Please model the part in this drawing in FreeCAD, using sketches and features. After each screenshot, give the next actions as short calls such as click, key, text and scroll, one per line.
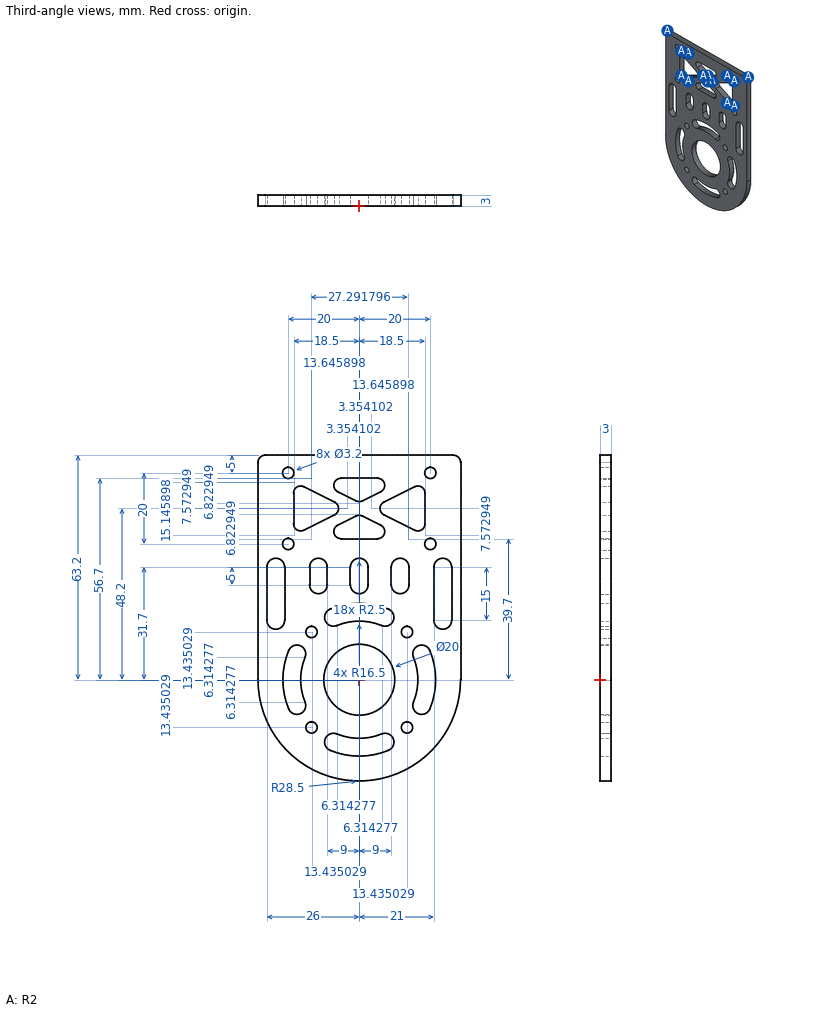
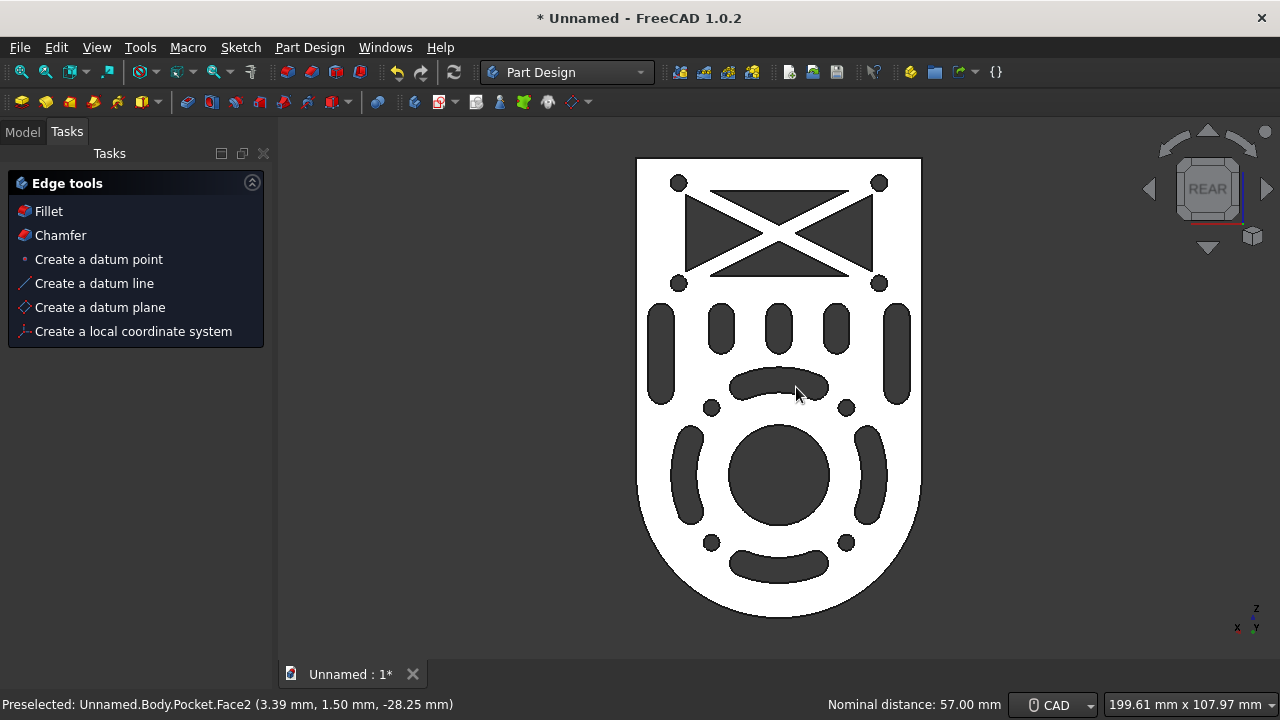
scroll(762, 232, up, 5)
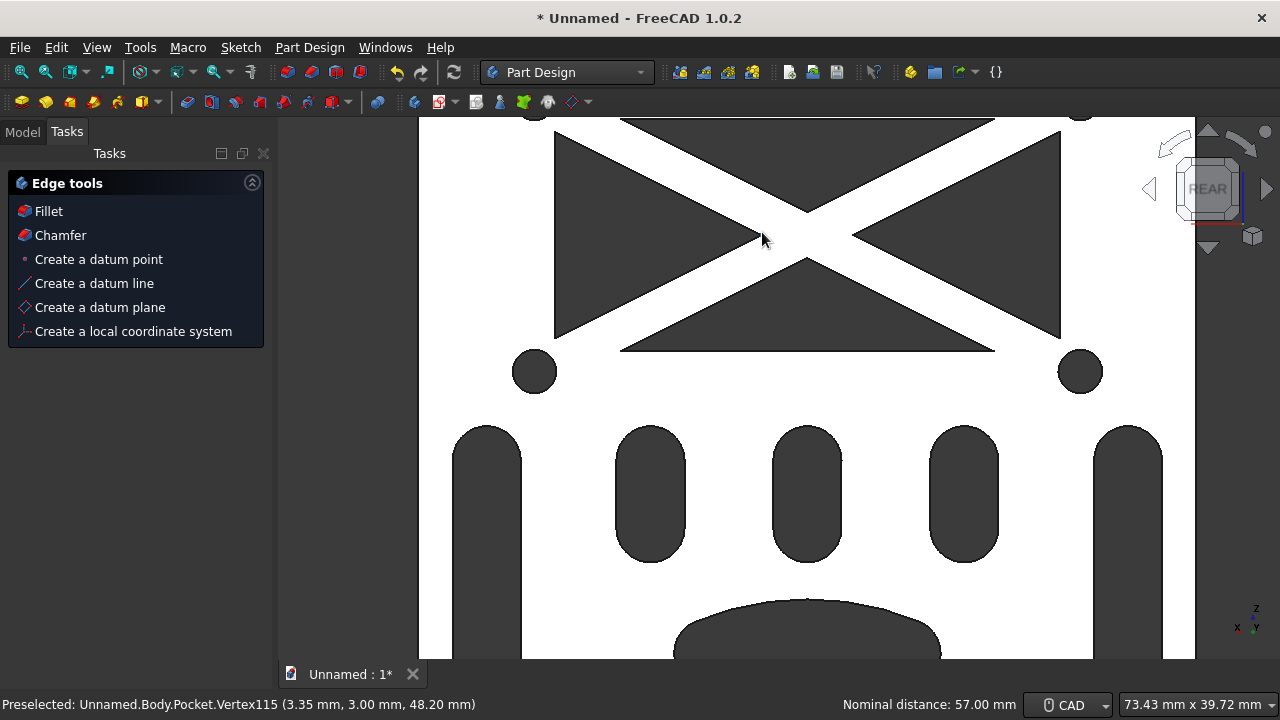
key(v)
key(f)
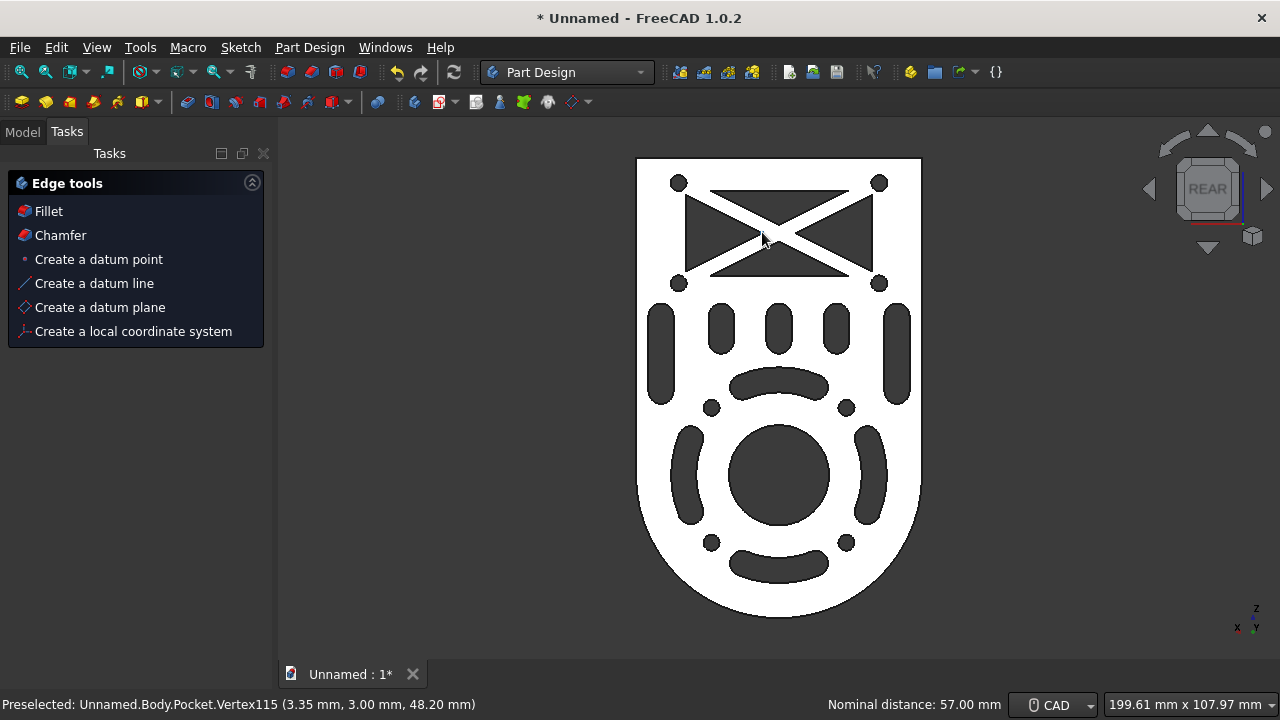
key(6)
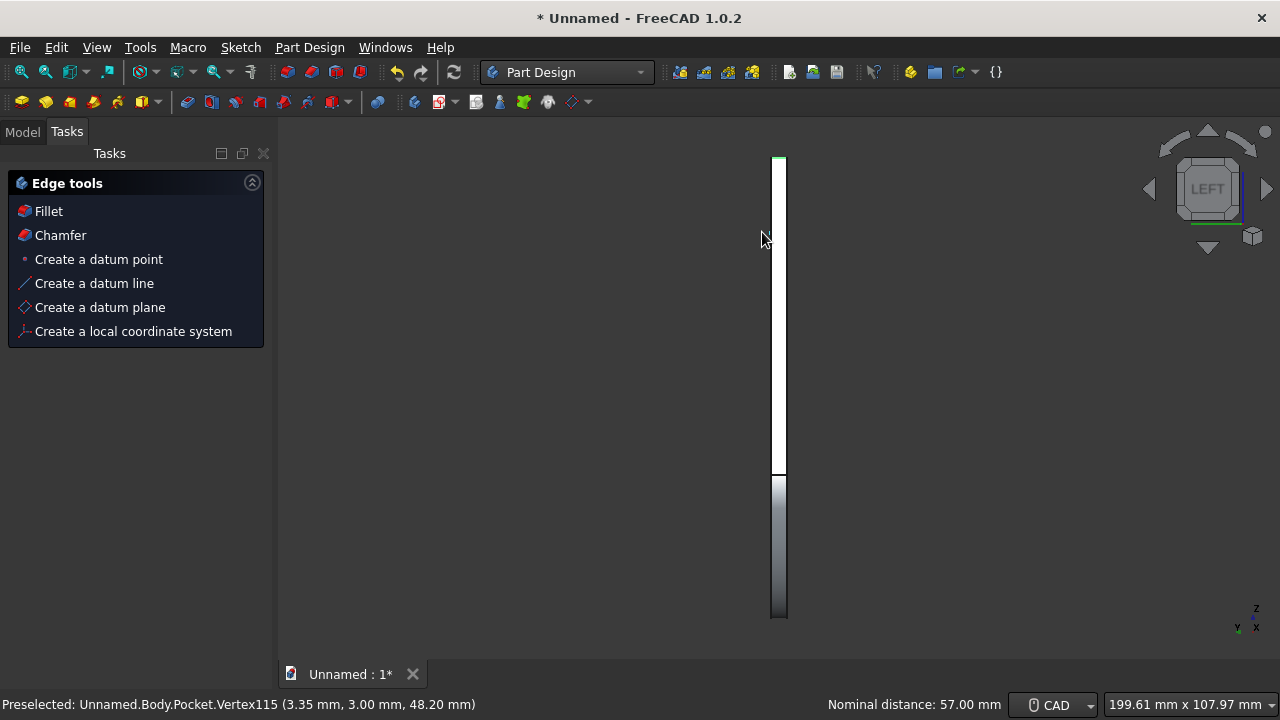
scroll(779, 232, up, 5)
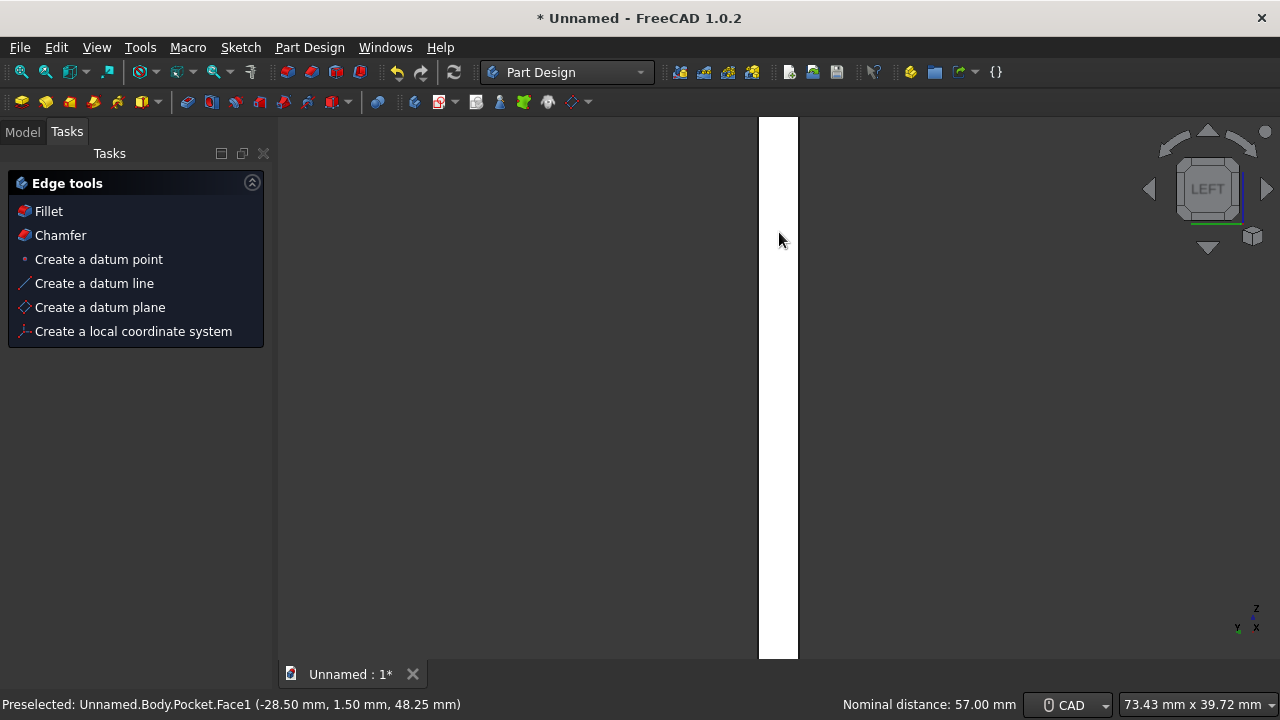
key(v)
key(f)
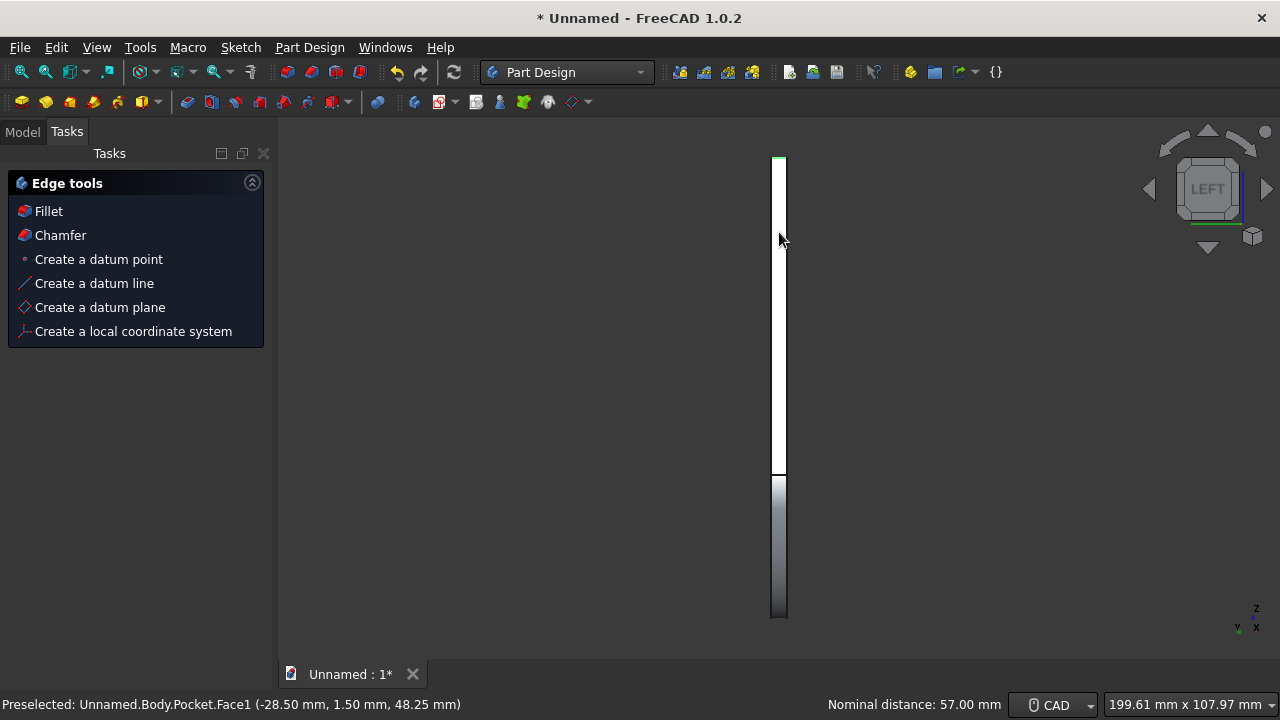
key(v)
key(3)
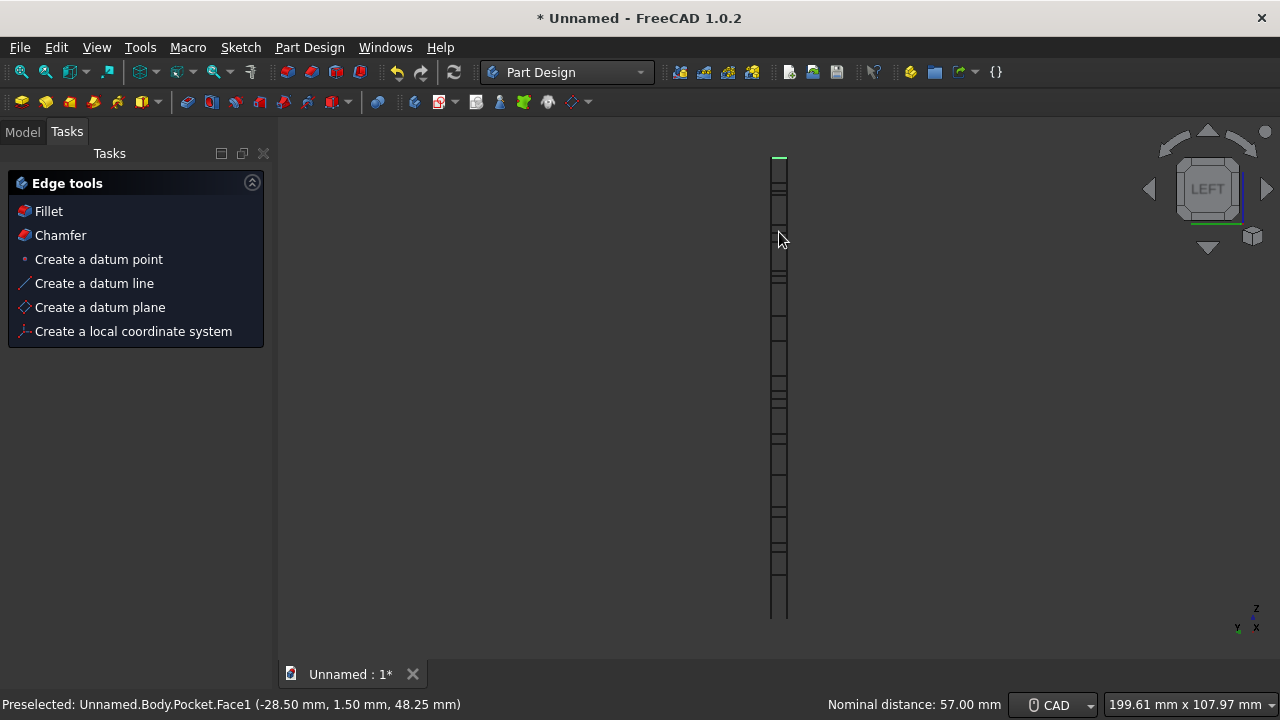
key(0)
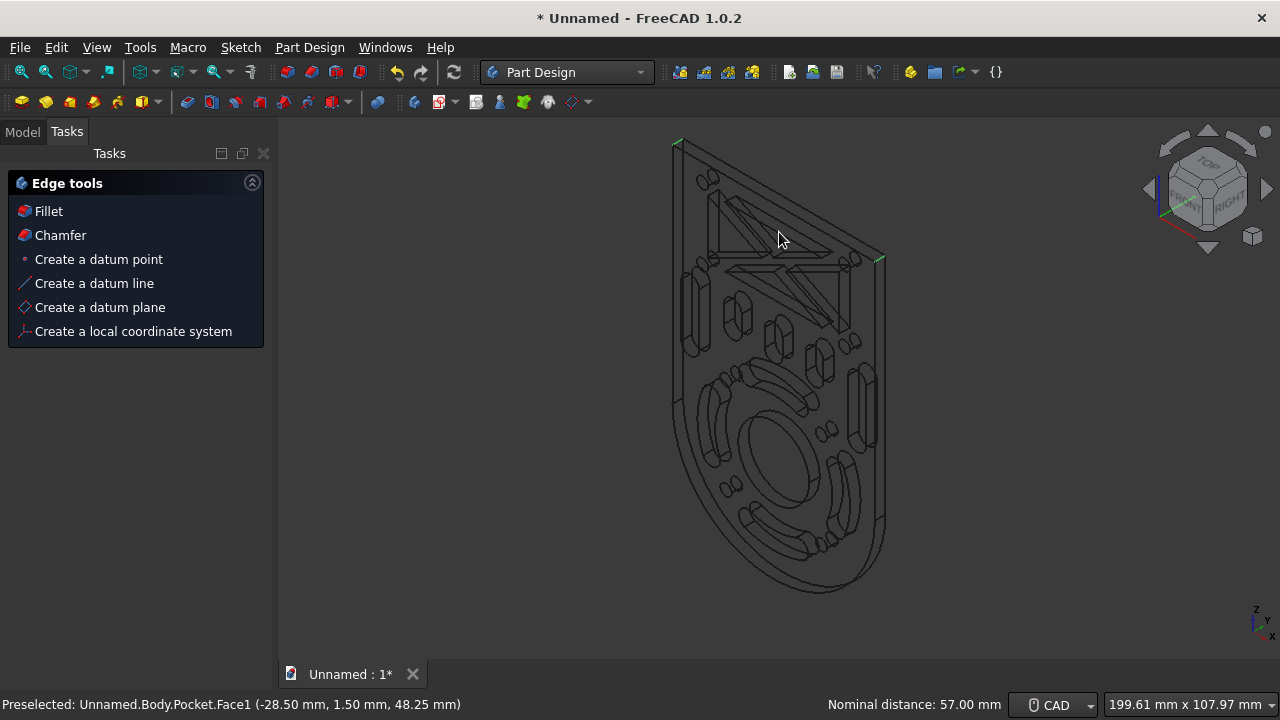
click(846, 329, ctrl)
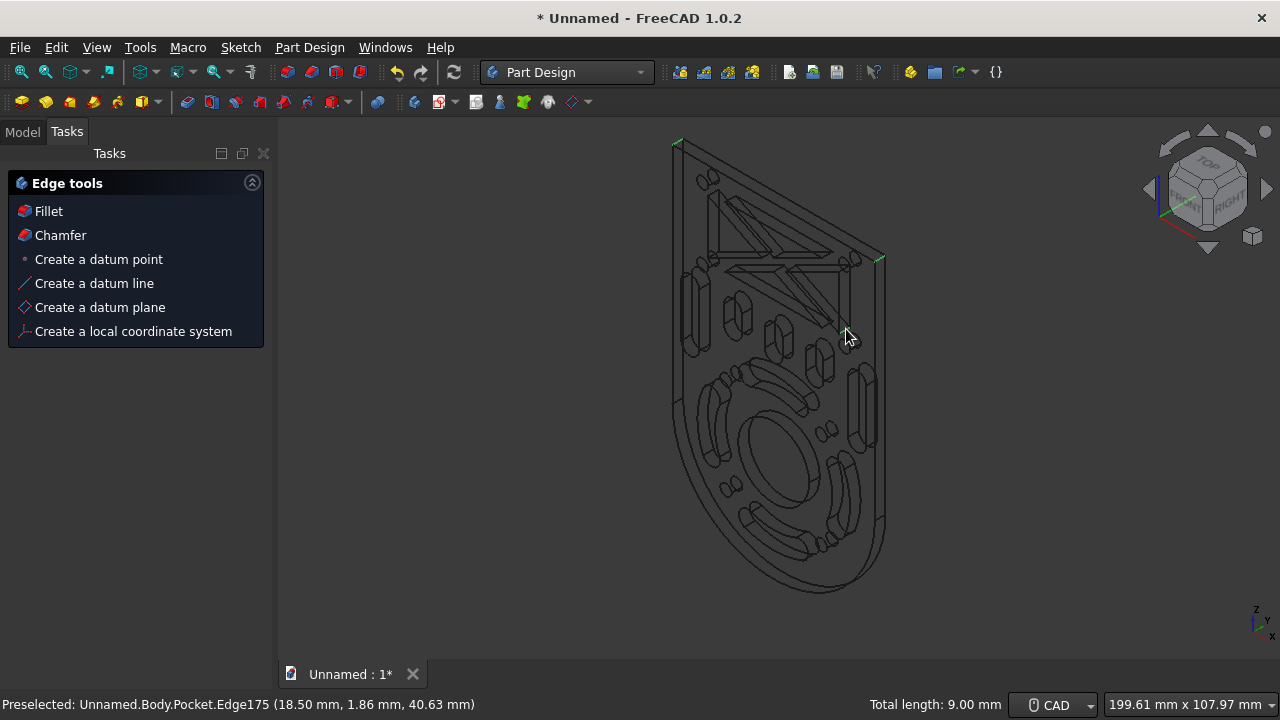
click(780, 267, ctrl)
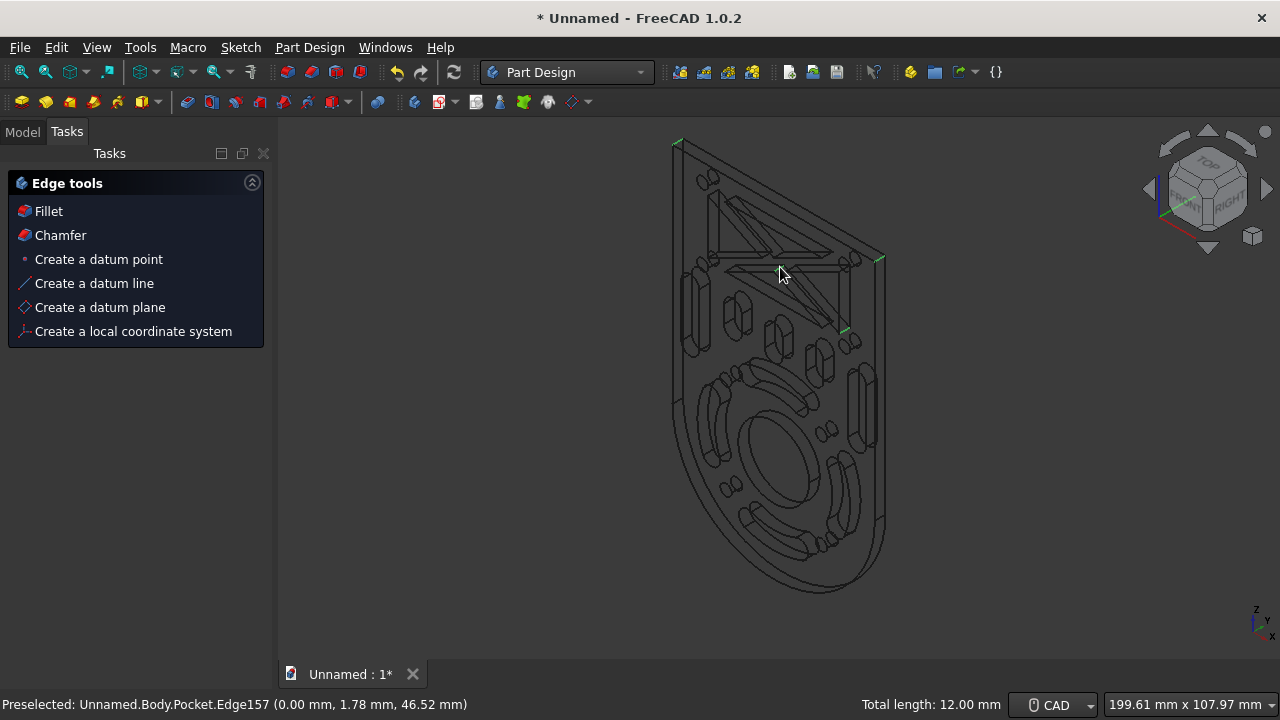
click(732, 197, ctrl)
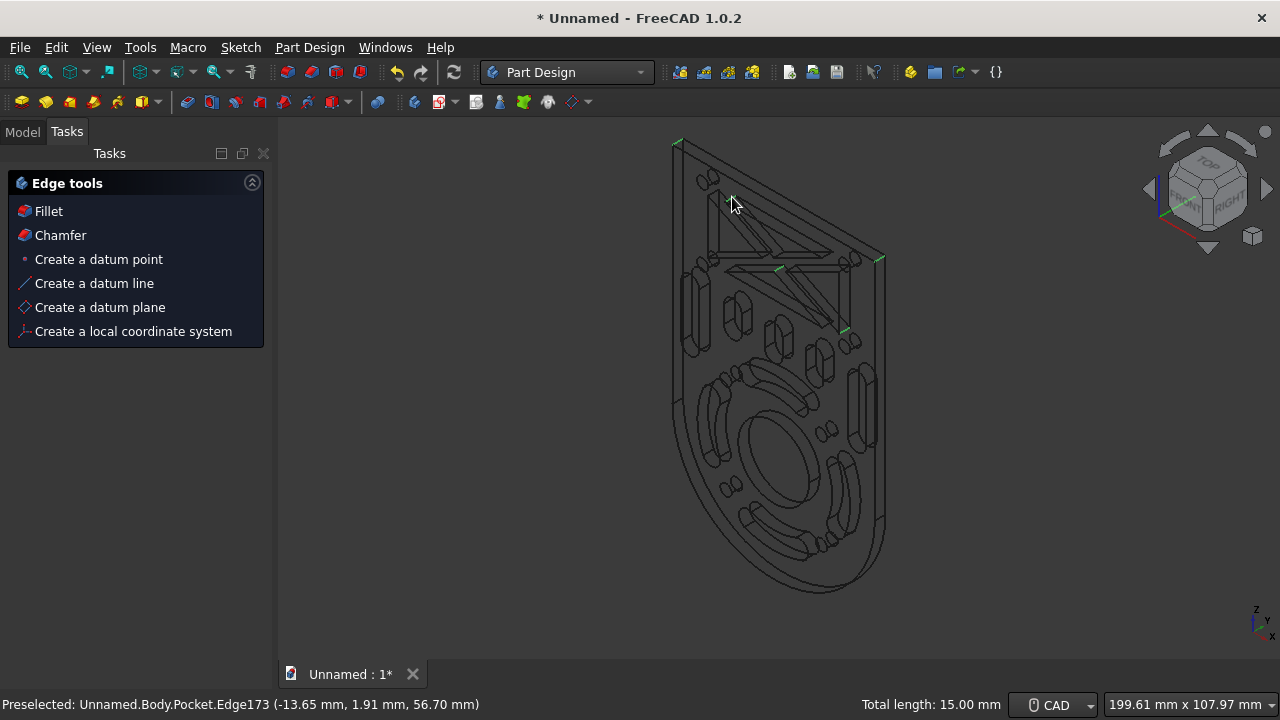
click(829, 253, ctrl)